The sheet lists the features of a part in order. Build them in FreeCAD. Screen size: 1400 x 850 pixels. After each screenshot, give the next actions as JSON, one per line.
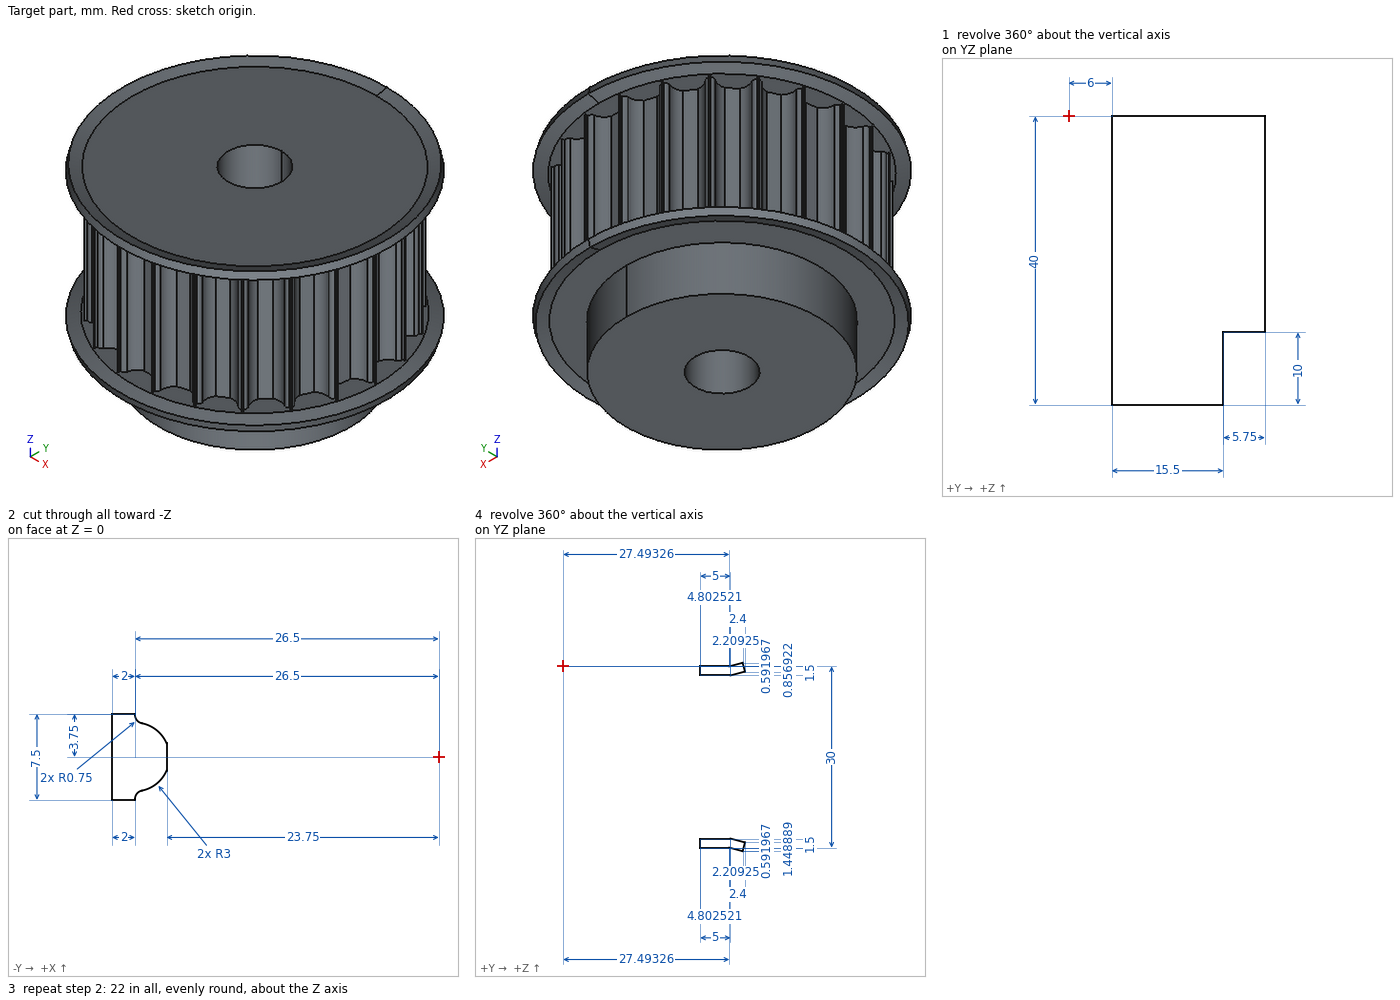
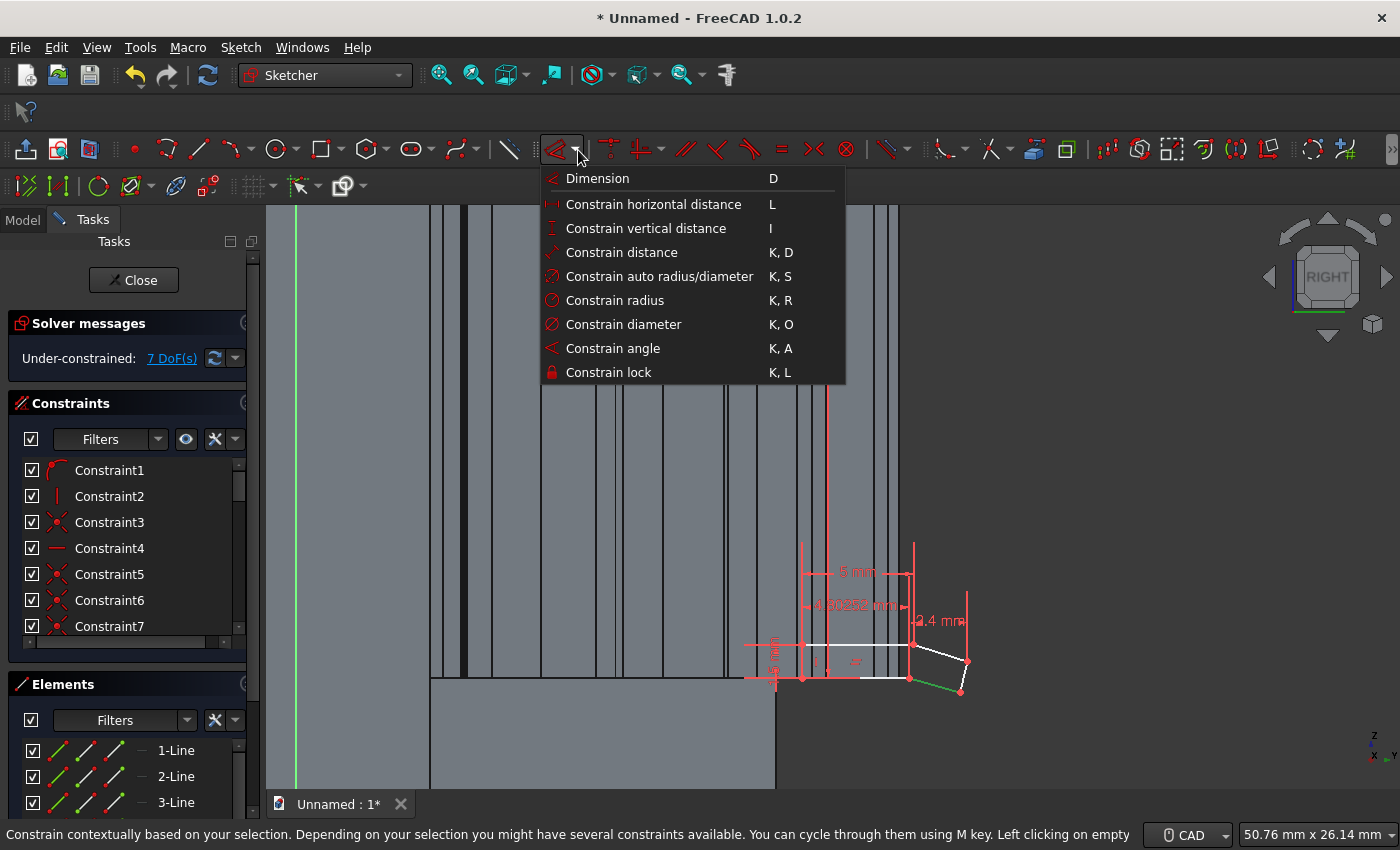
{"action": "left_click", "coordinate": [693, 204]}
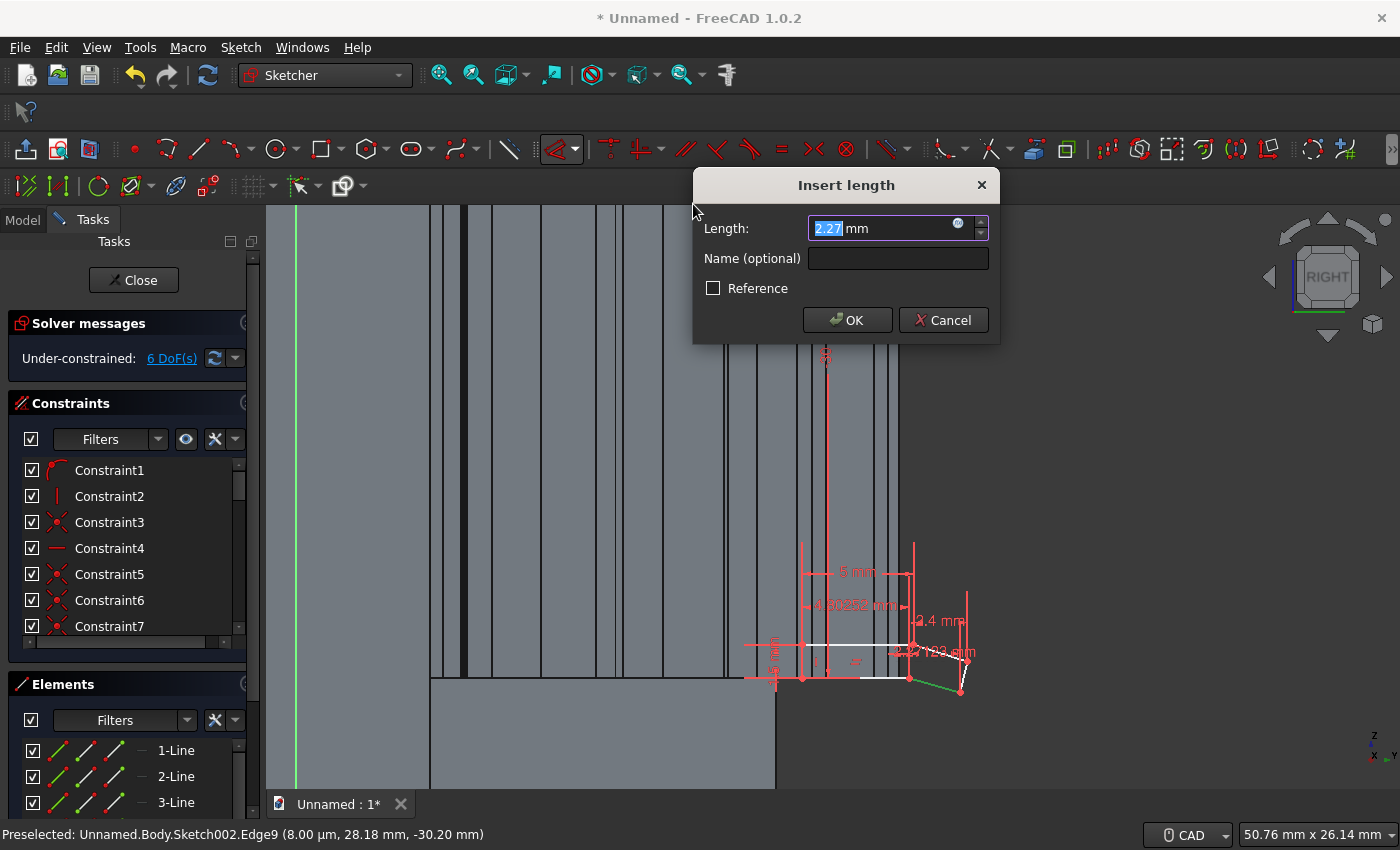
{"action": "type", "text": "2.20925"}
{"action": "key", "text": "Return"}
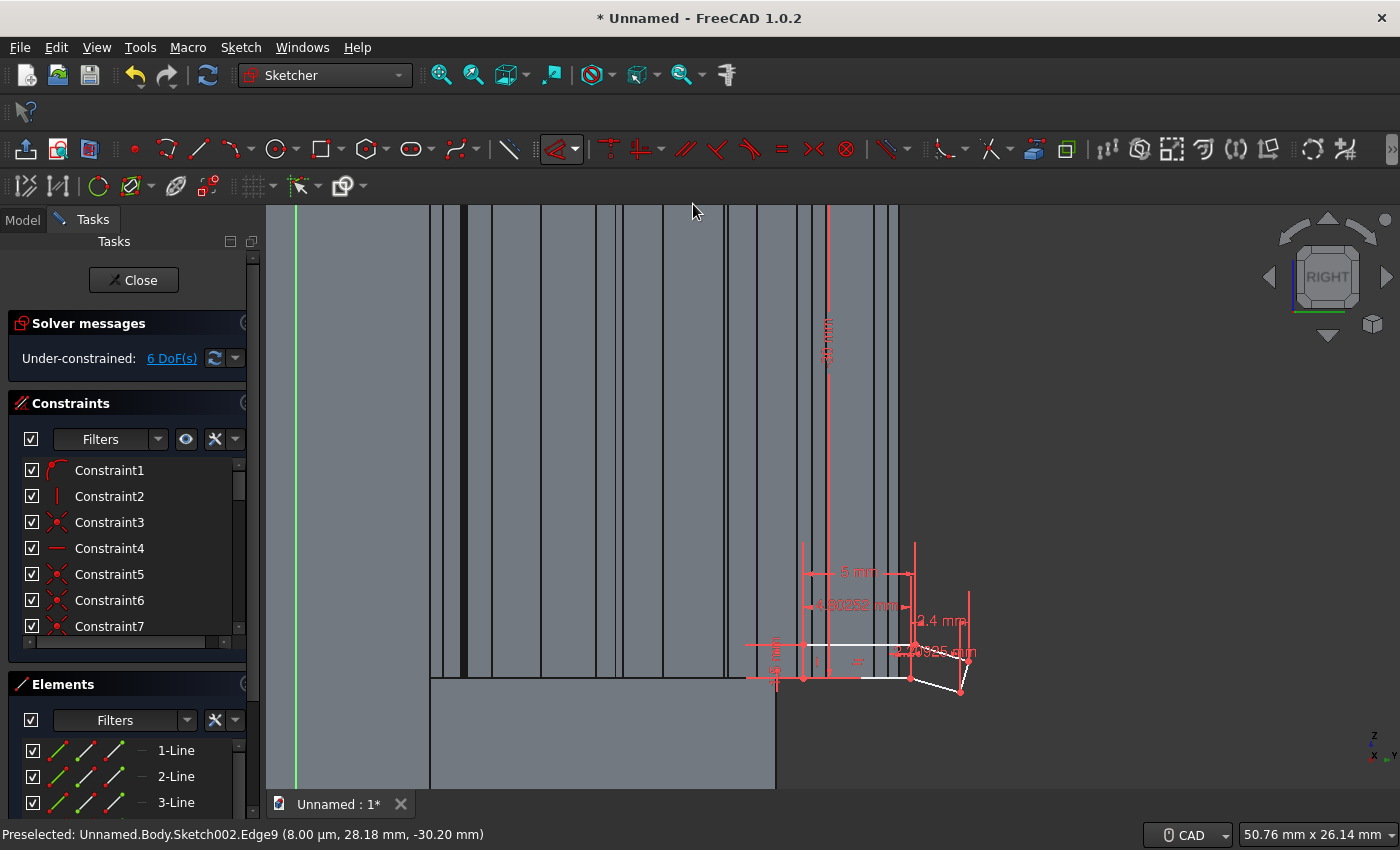
{"action": "scroll", "coordinate": [926, 684], "scroll_direction": "down", "scroll_amount": 3}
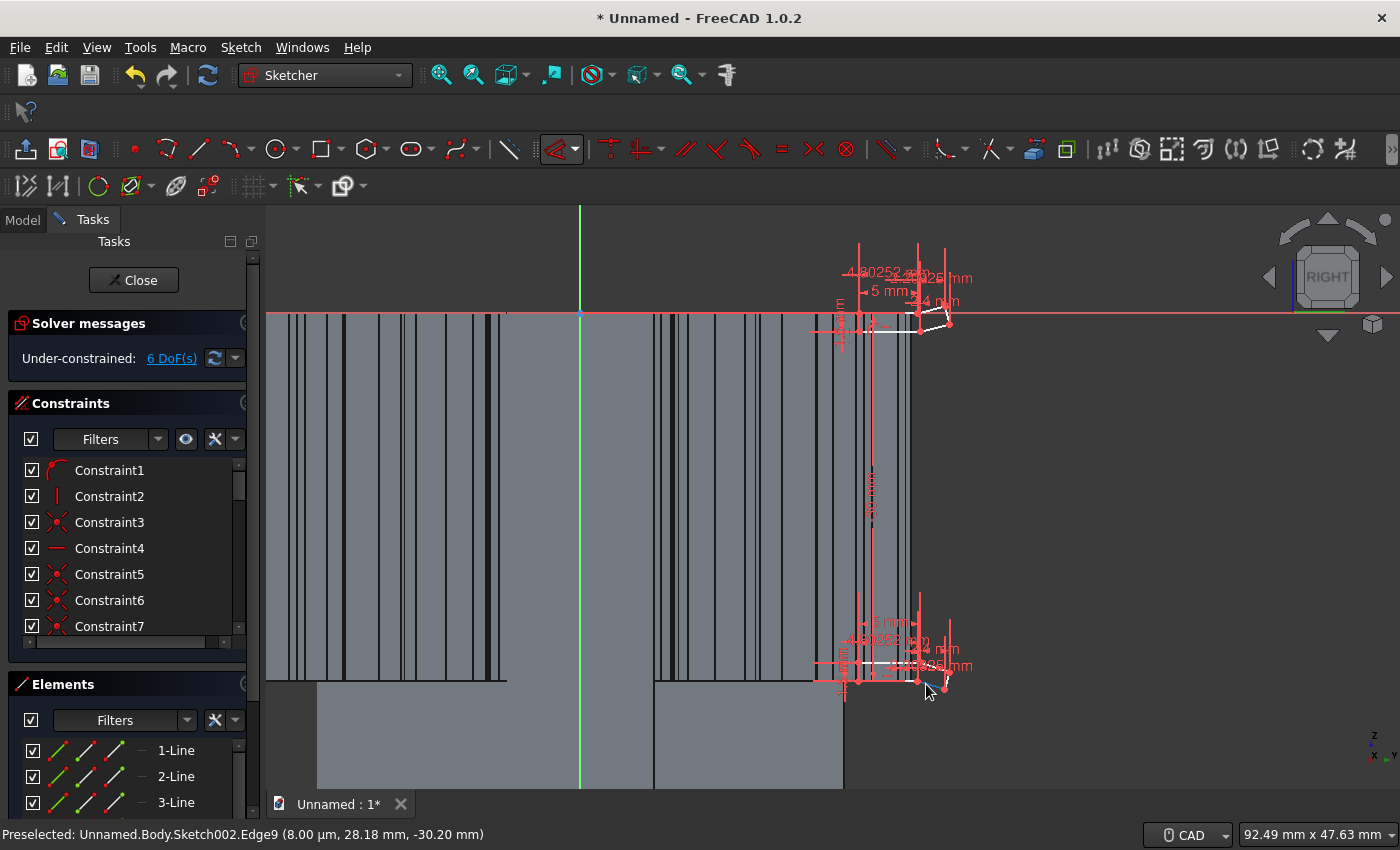
{"action": "scroll", "coordinate": [950, 325], "scroll_direction": "up", "scroll_amount": 7}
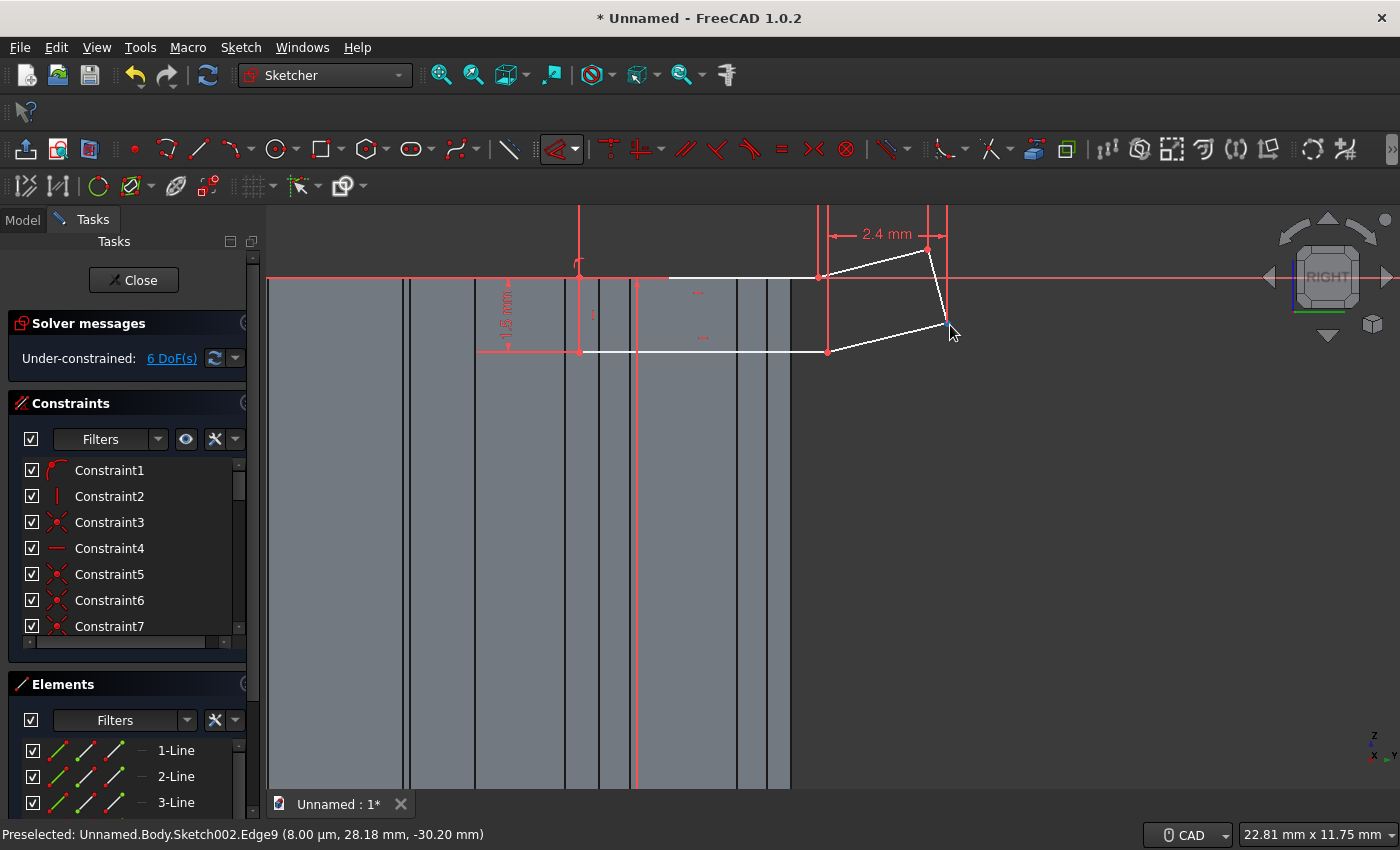
{"action": "left_click", "coordinate": [947, 323]}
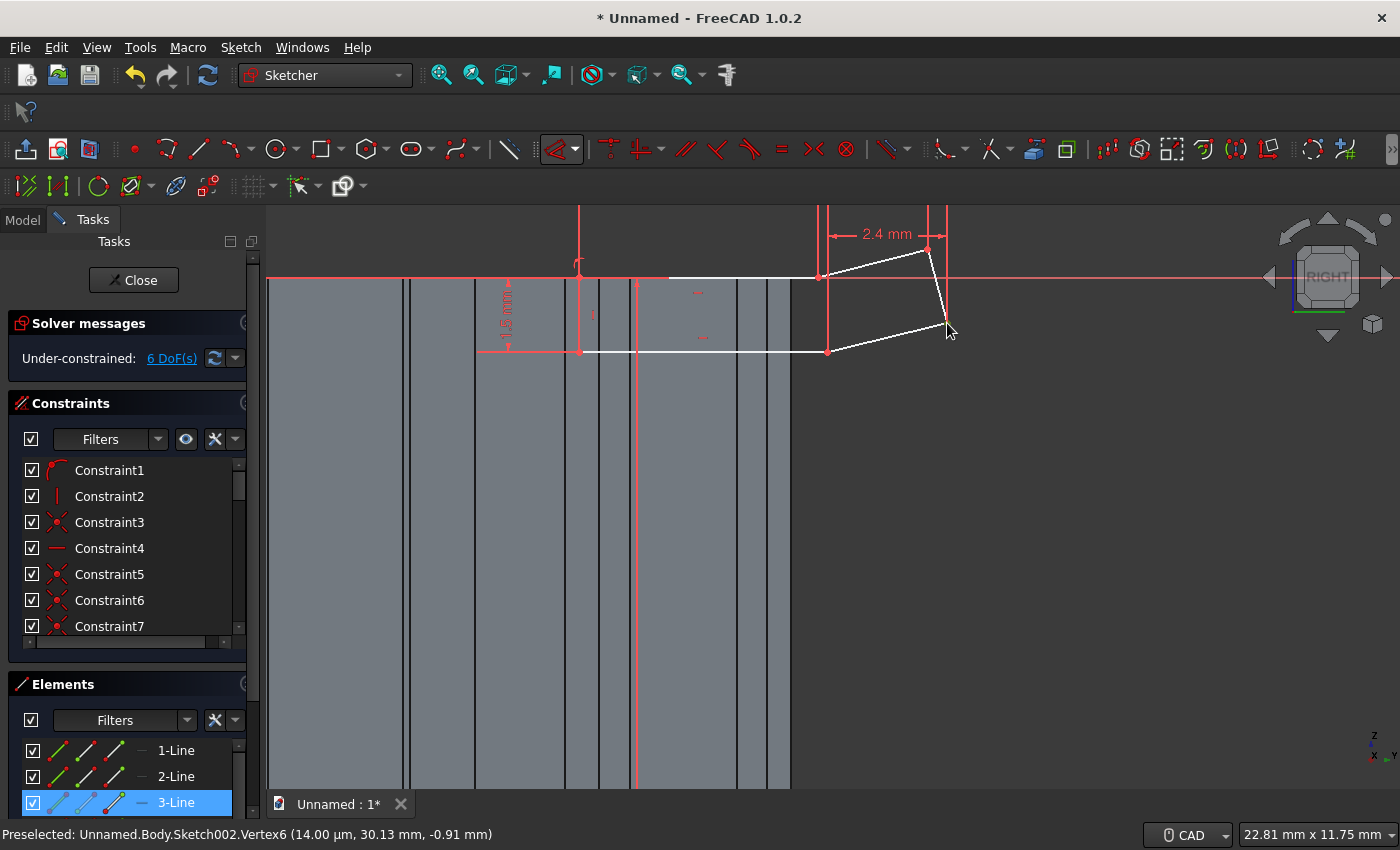
{"action": "left_click", "coordinate": [578, 150]}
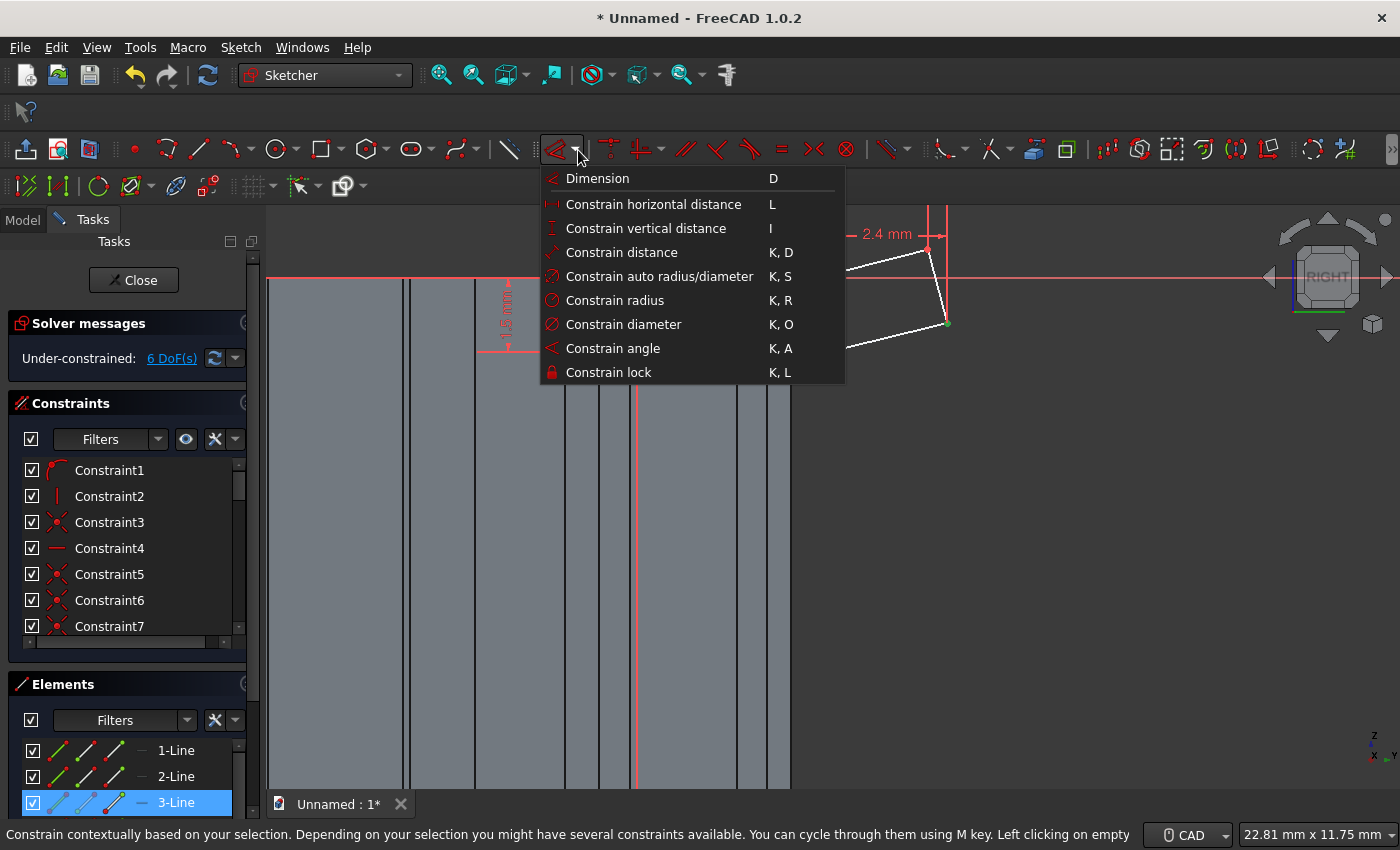
{"action": "left_click", "coordinate": [693, 228]}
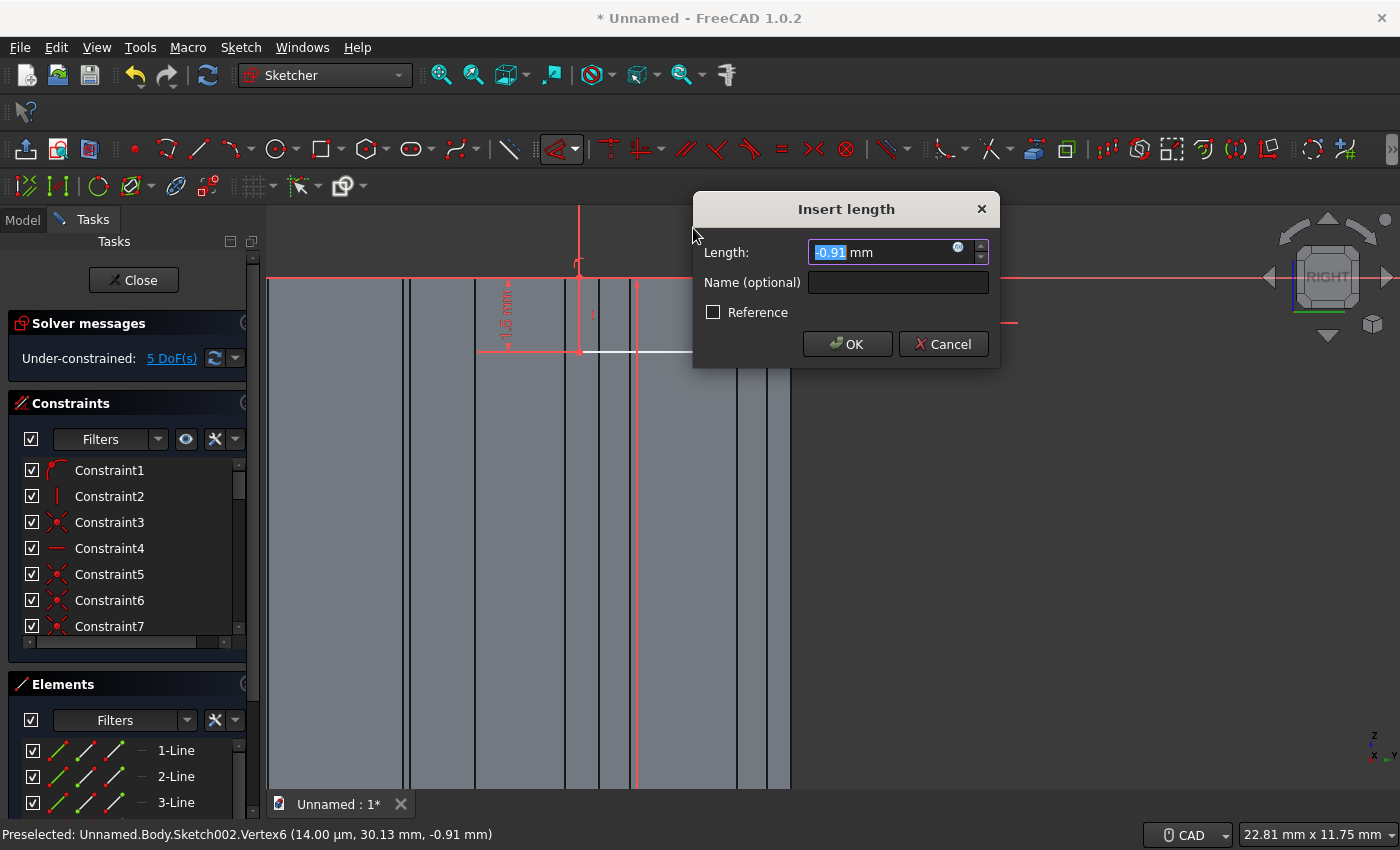
{"action": "type", "text": "-0.856922"}
{"action": "key", "text": "Return"}